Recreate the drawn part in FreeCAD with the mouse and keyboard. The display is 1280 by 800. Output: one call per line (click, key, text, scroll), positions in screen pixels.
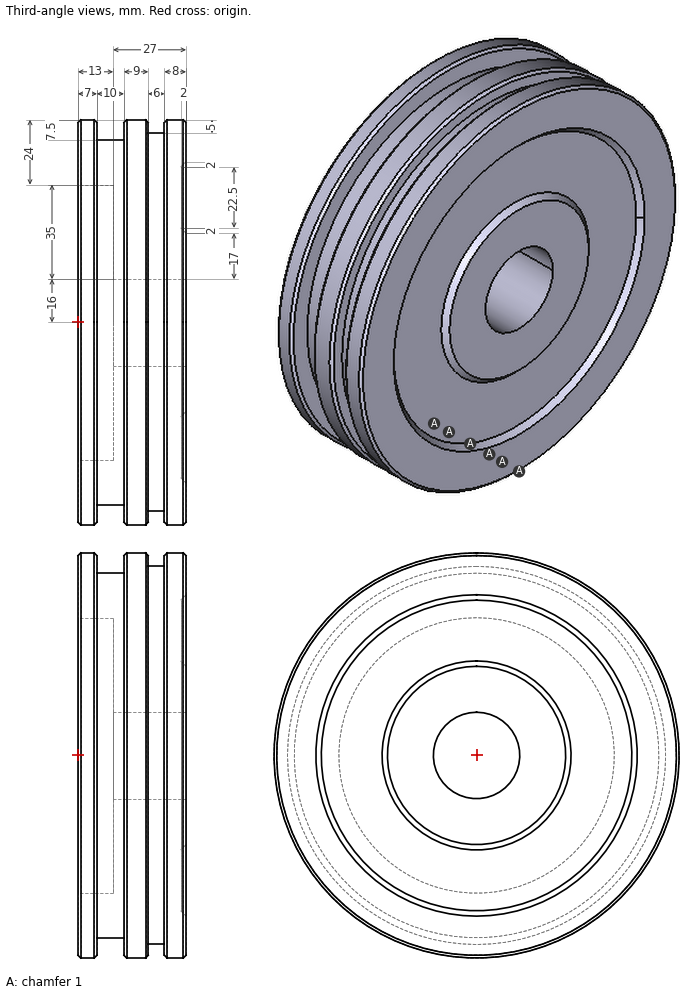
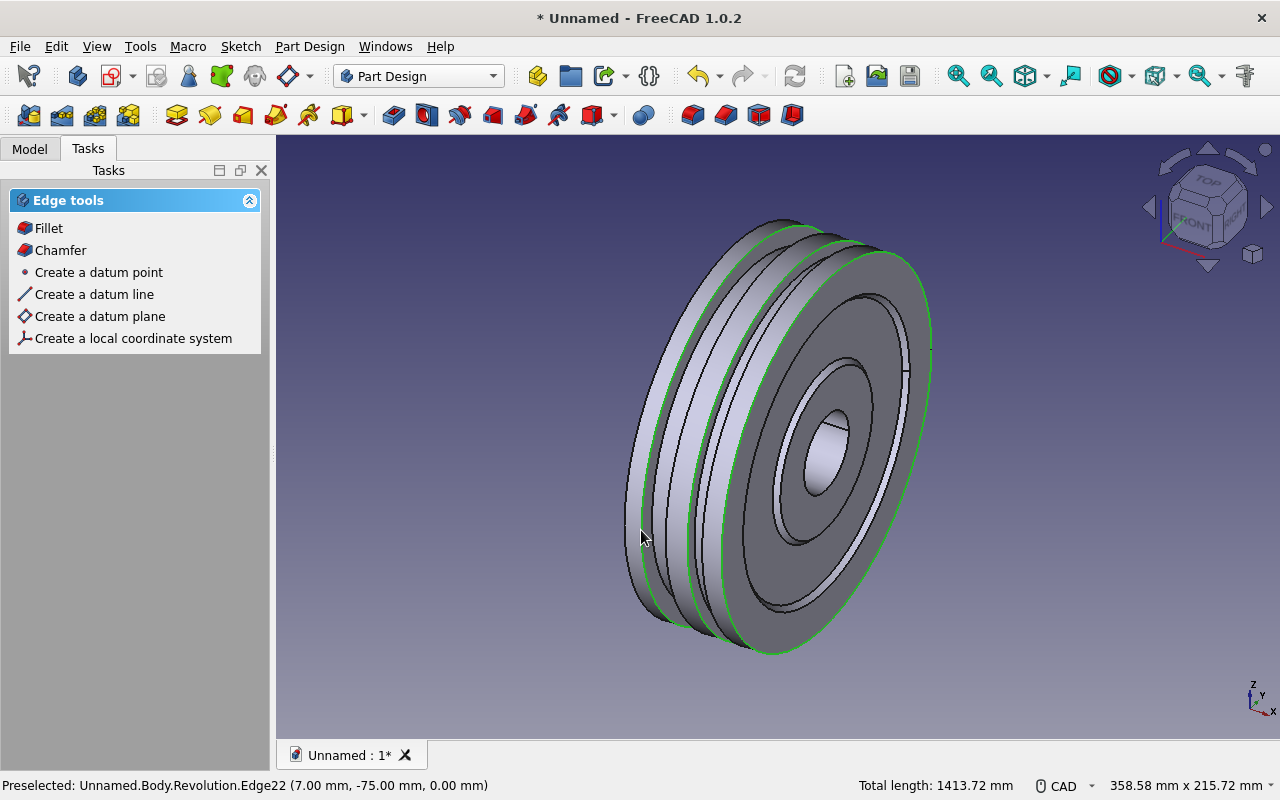
key(0)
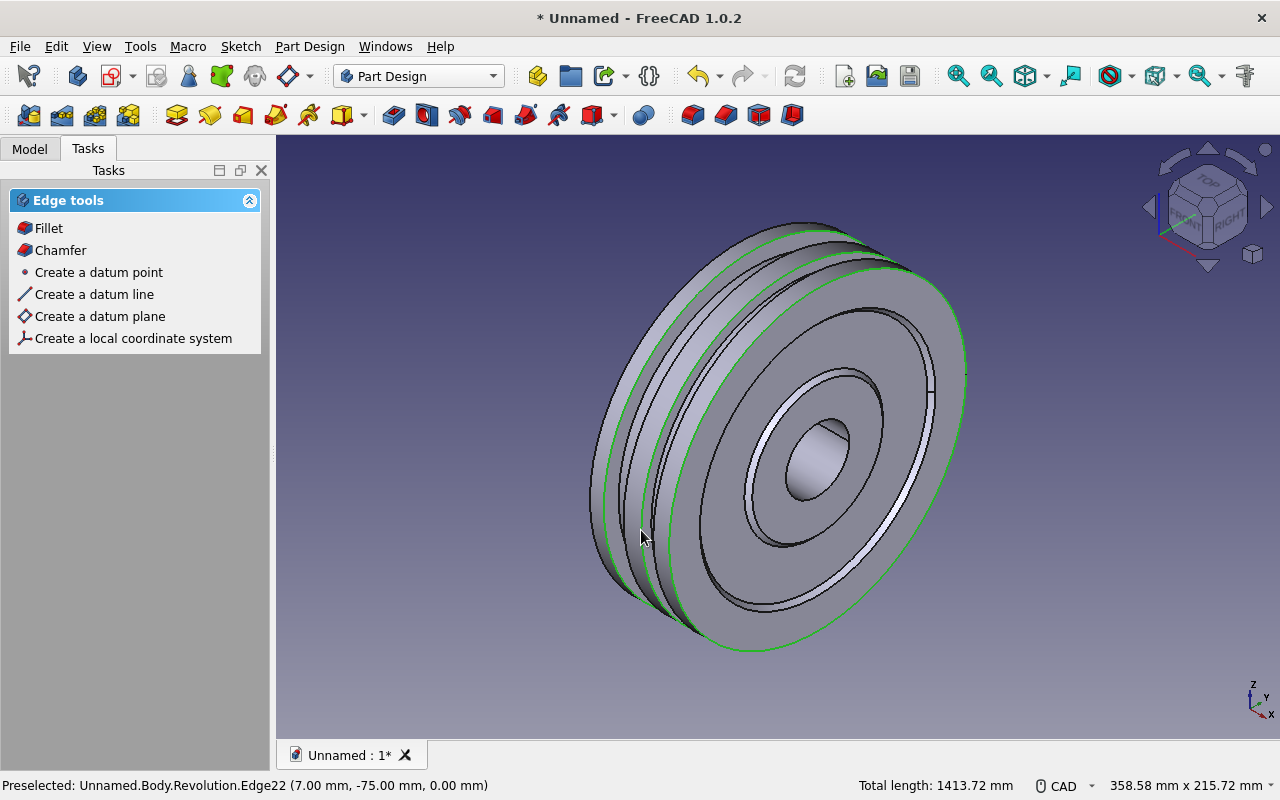
key(2)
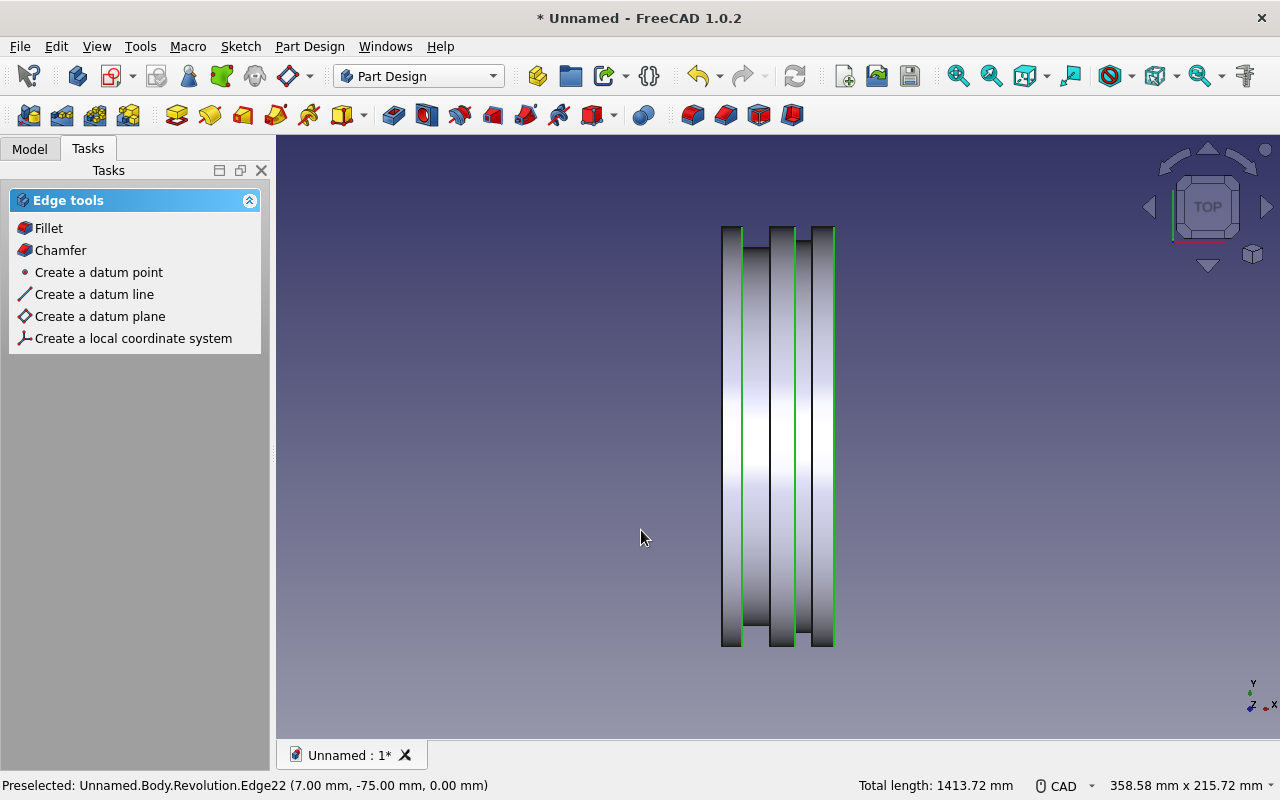
click(812, 606, ctrl)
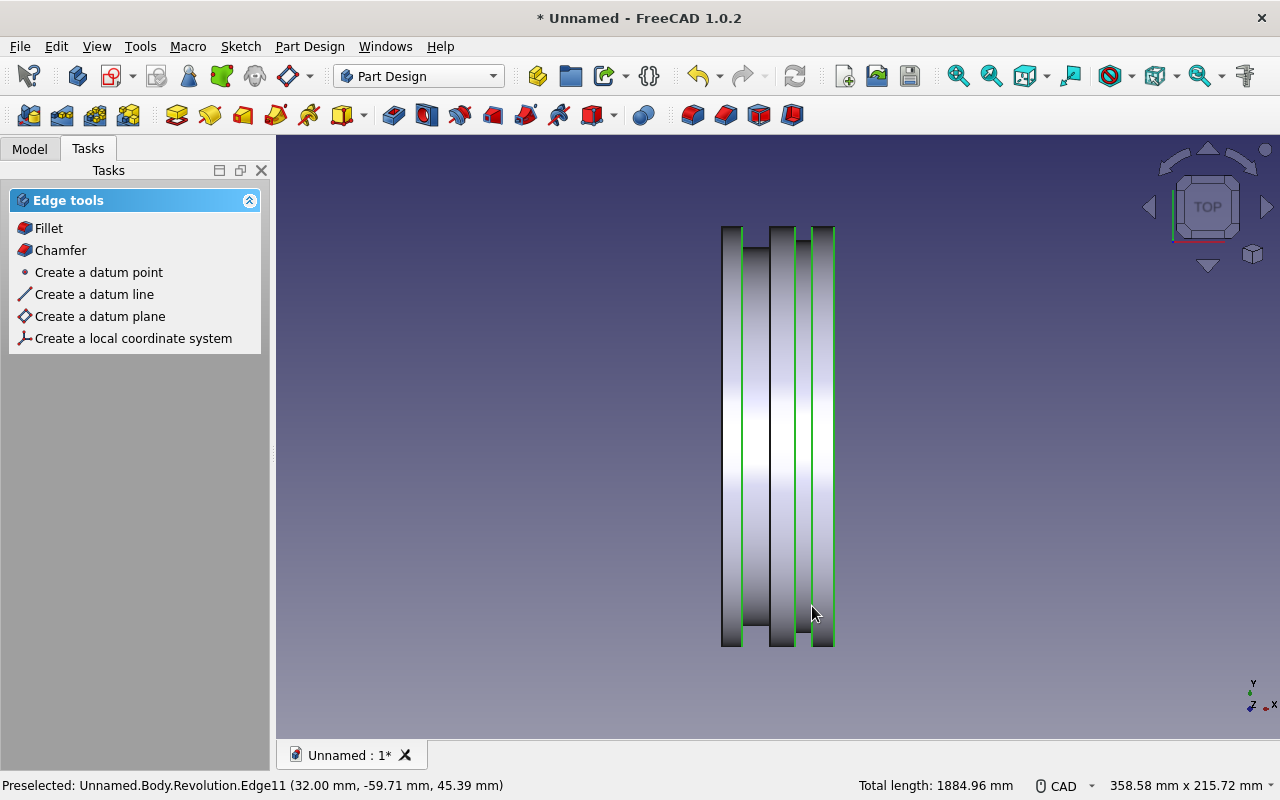
click(770, 606, ctrl)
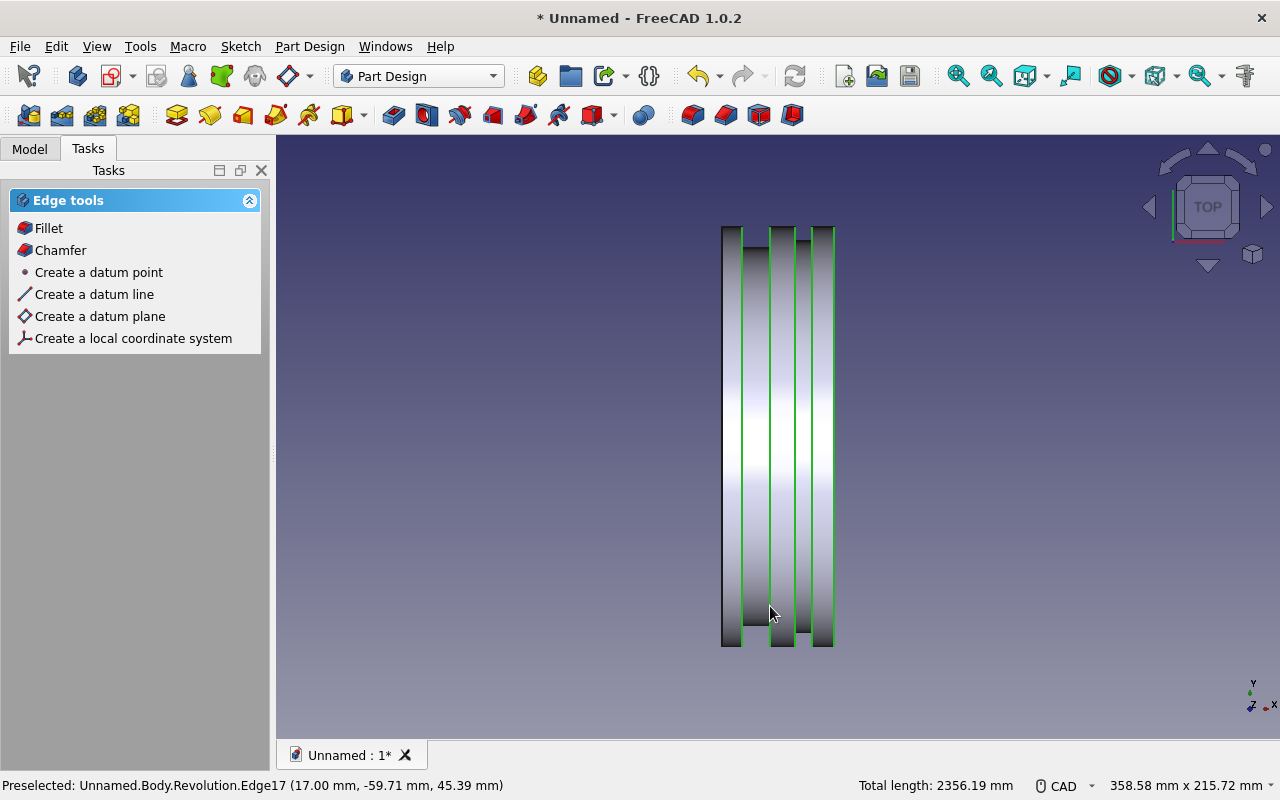
click(722, 606, ctrl)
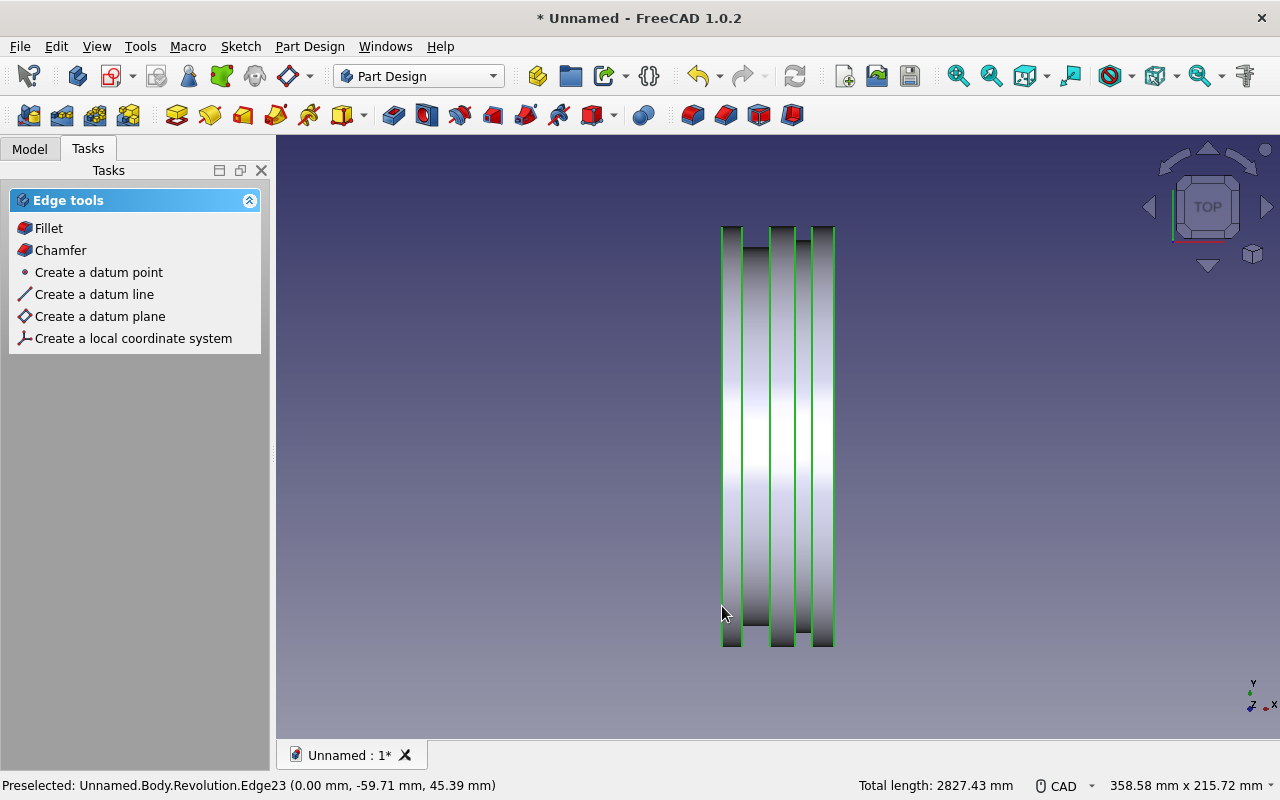
click(726, 116)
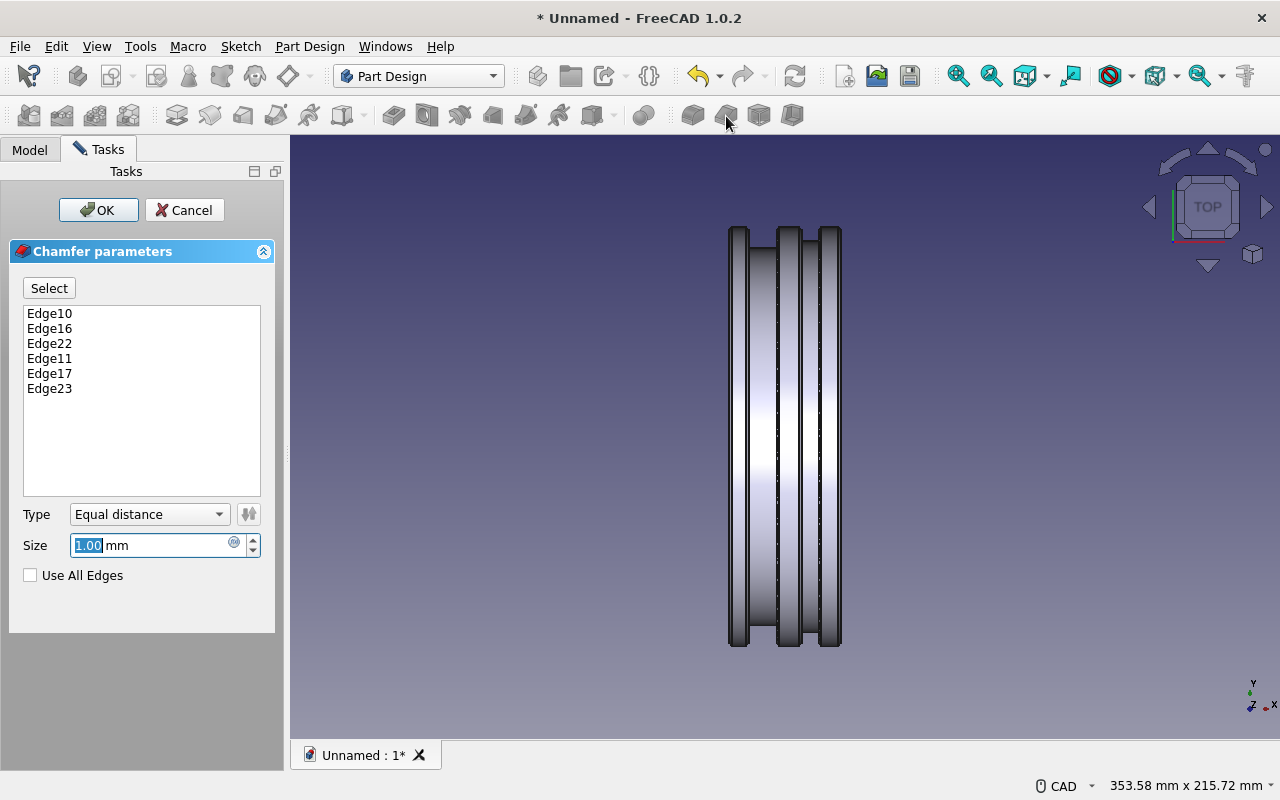
text(1)
key(Tab)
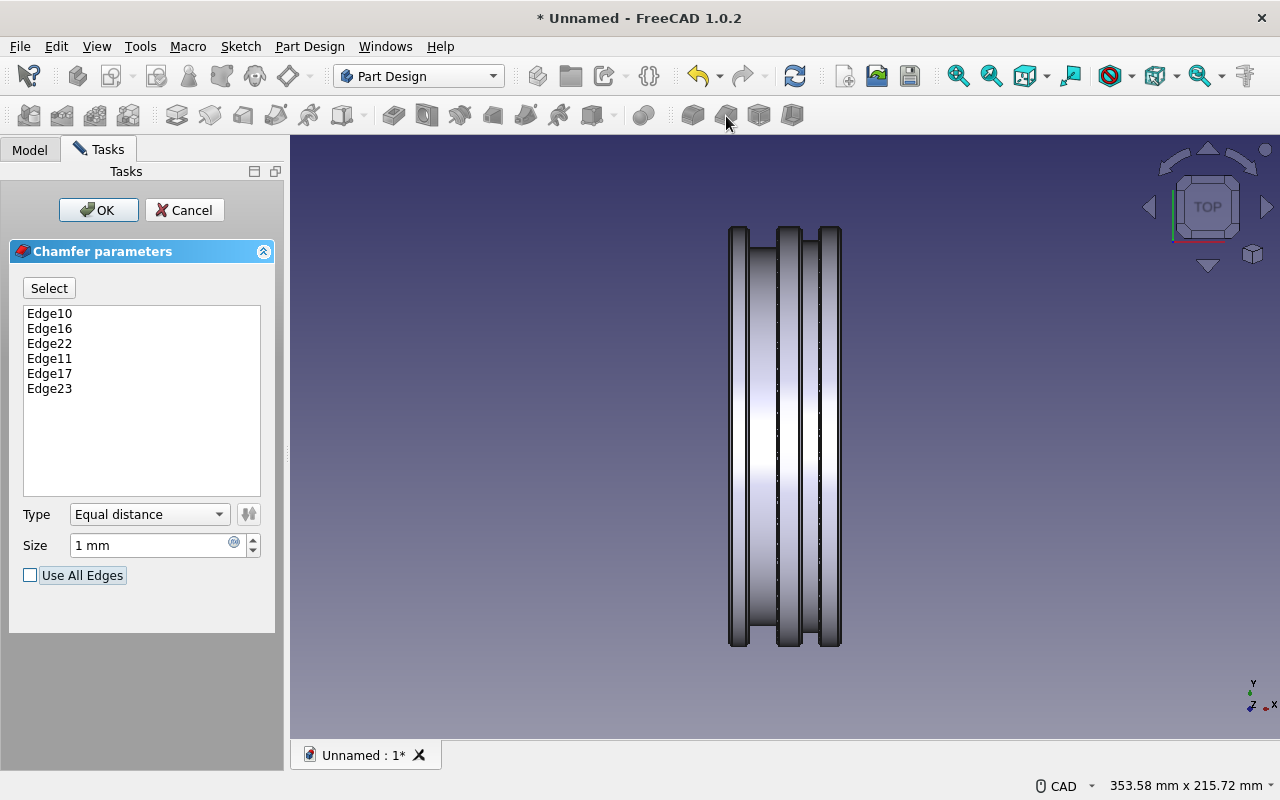
click(99, 210)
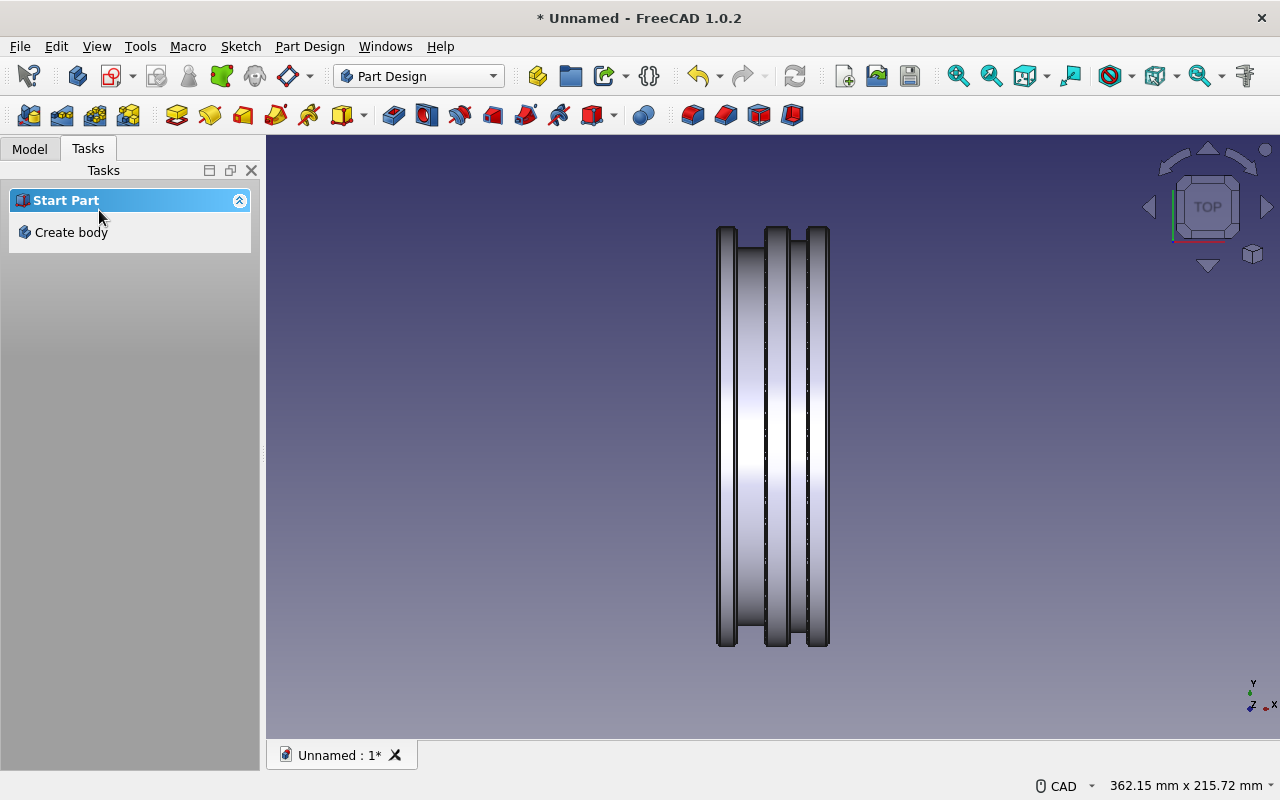
key(0)